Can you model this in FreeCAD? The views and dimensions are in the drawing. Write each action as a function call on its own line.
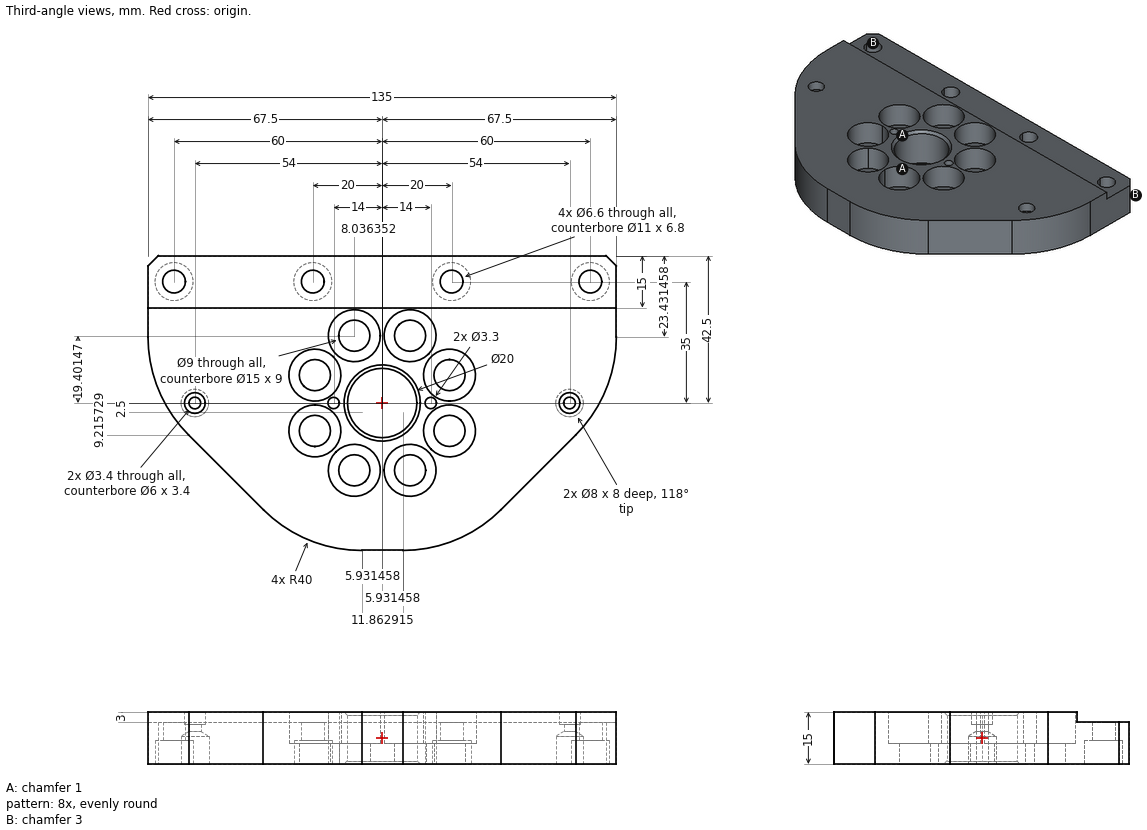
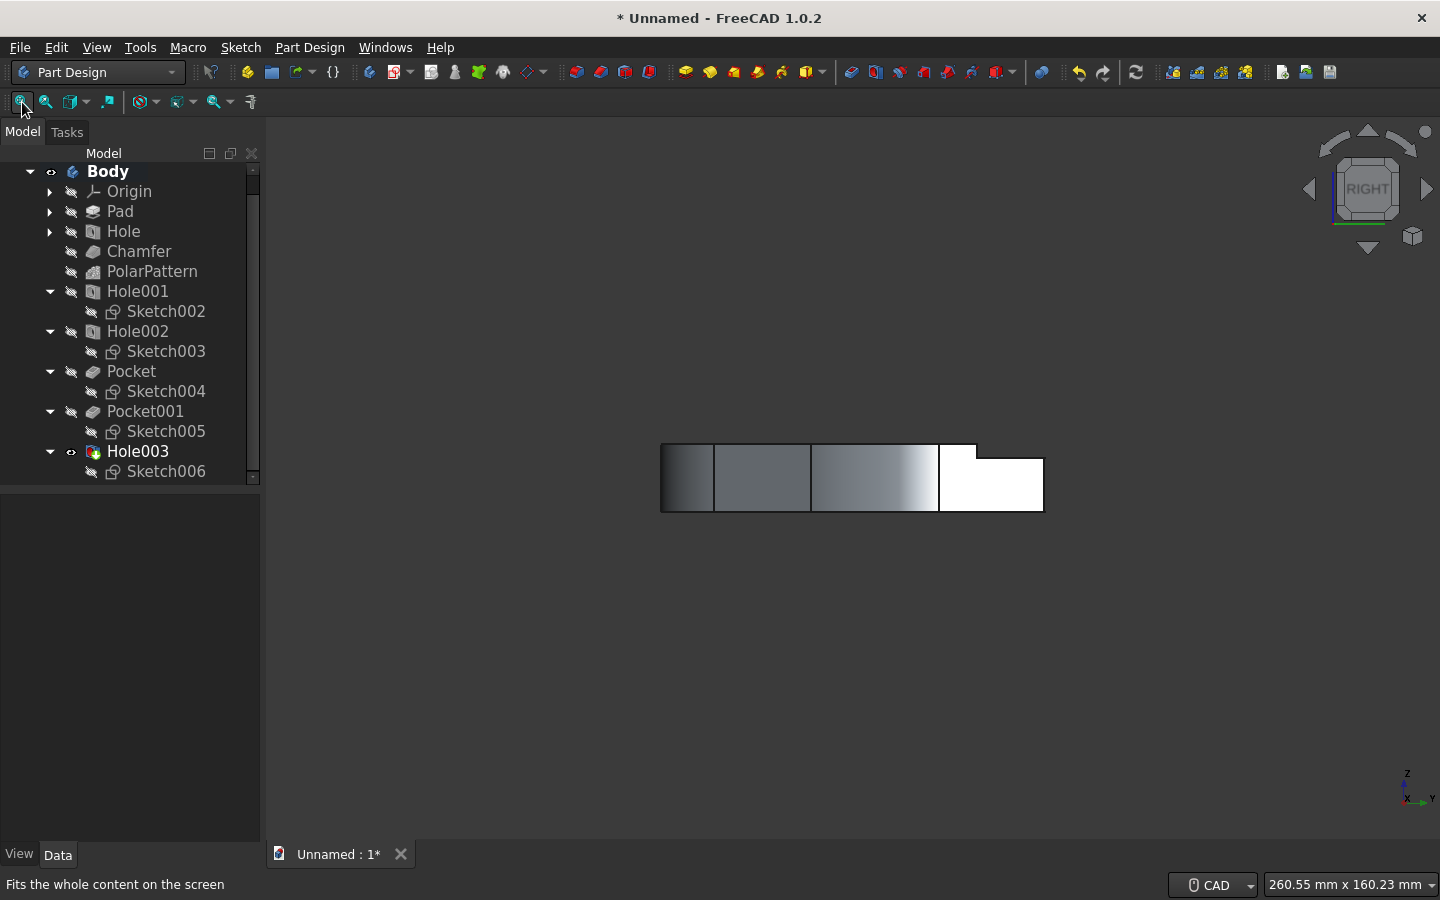
click(1045, 484)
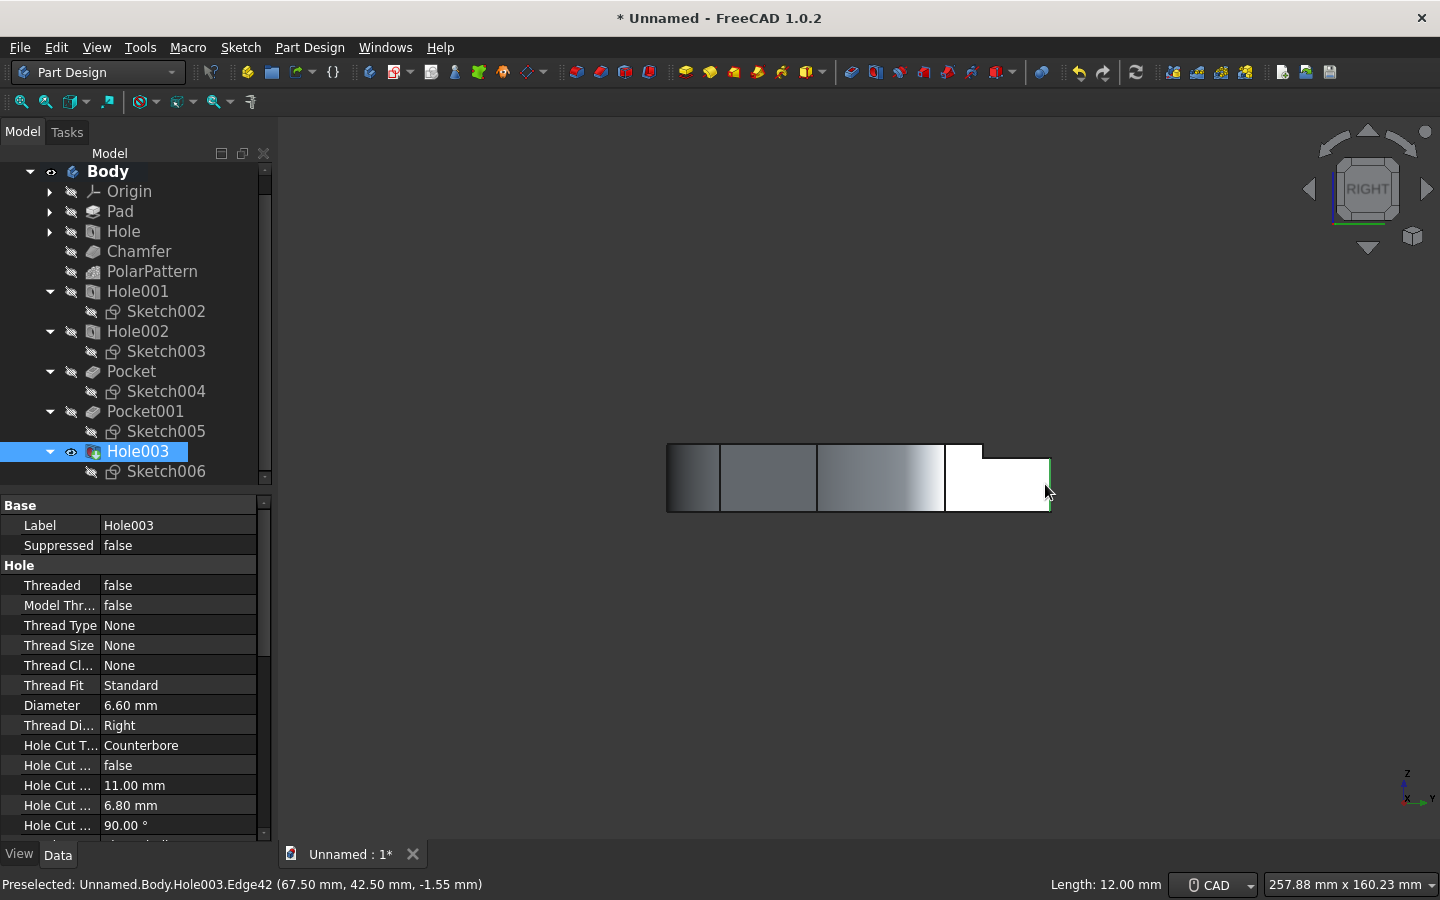
key(5)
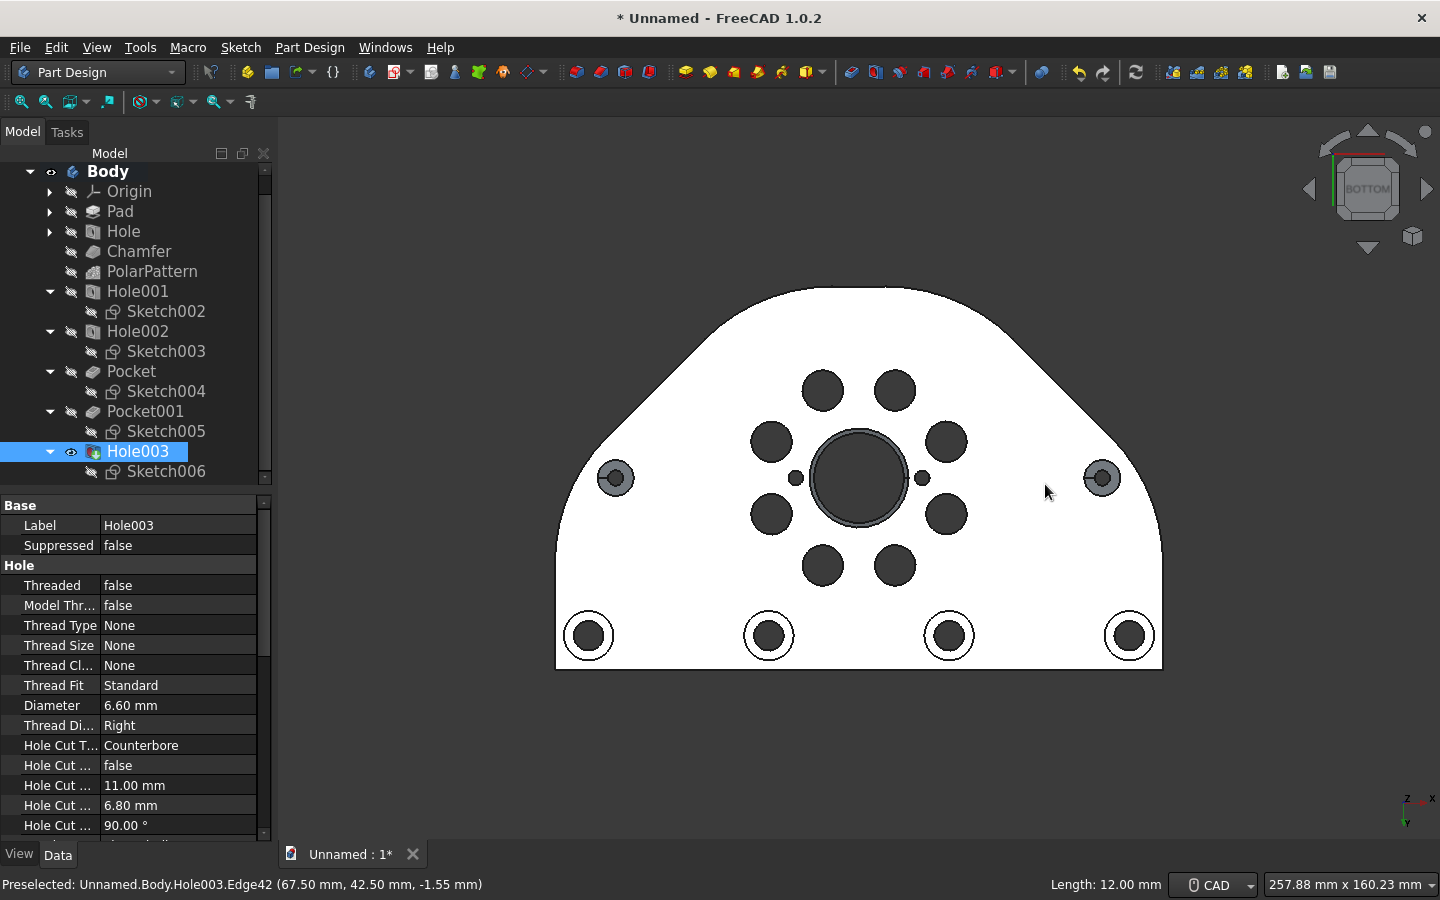
key(4)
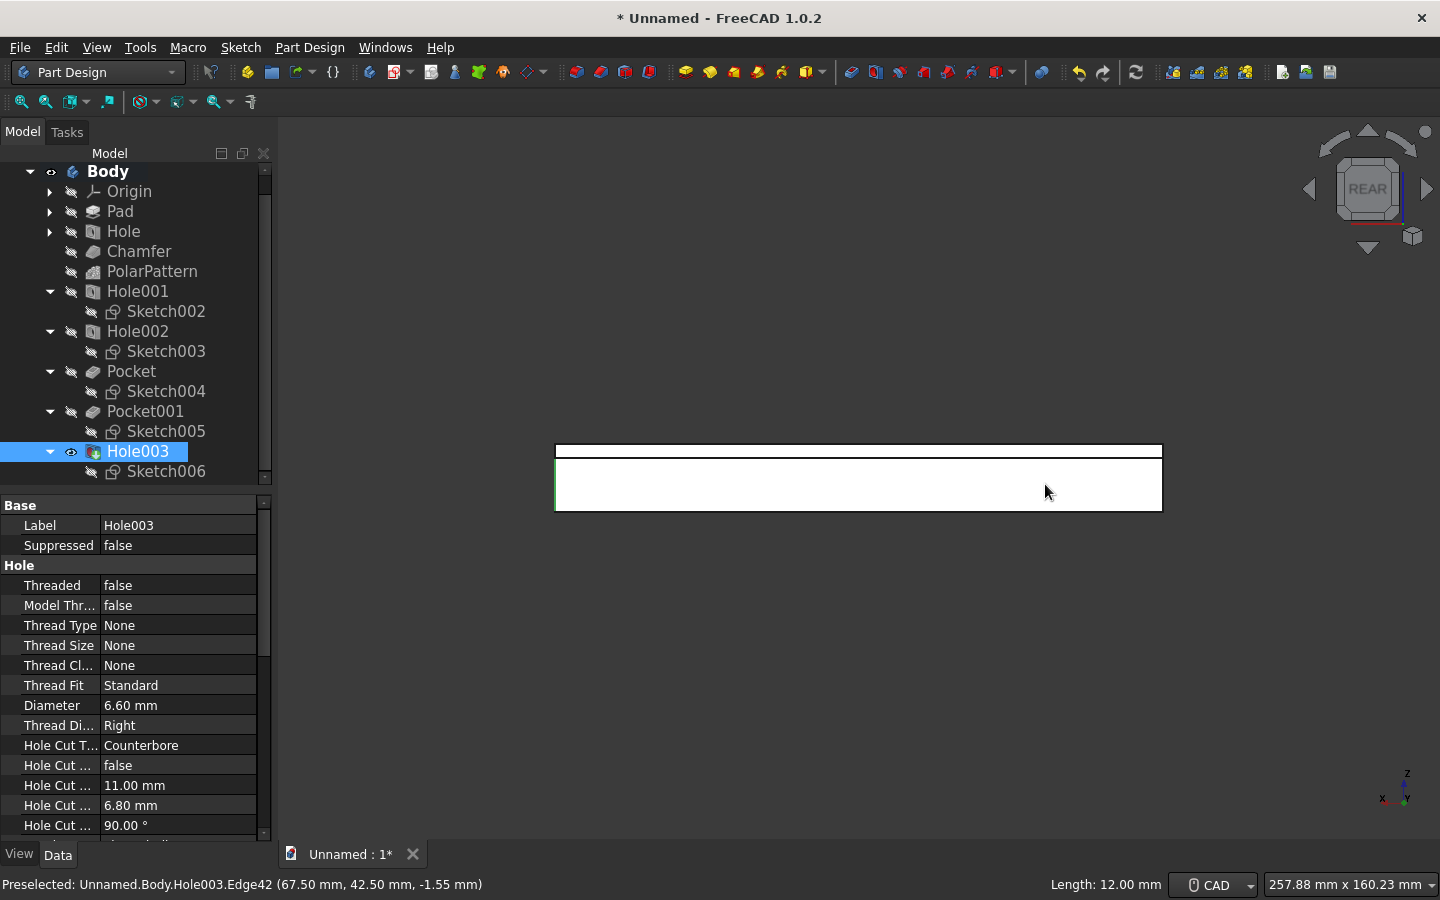
click(1163, 484, ctrl)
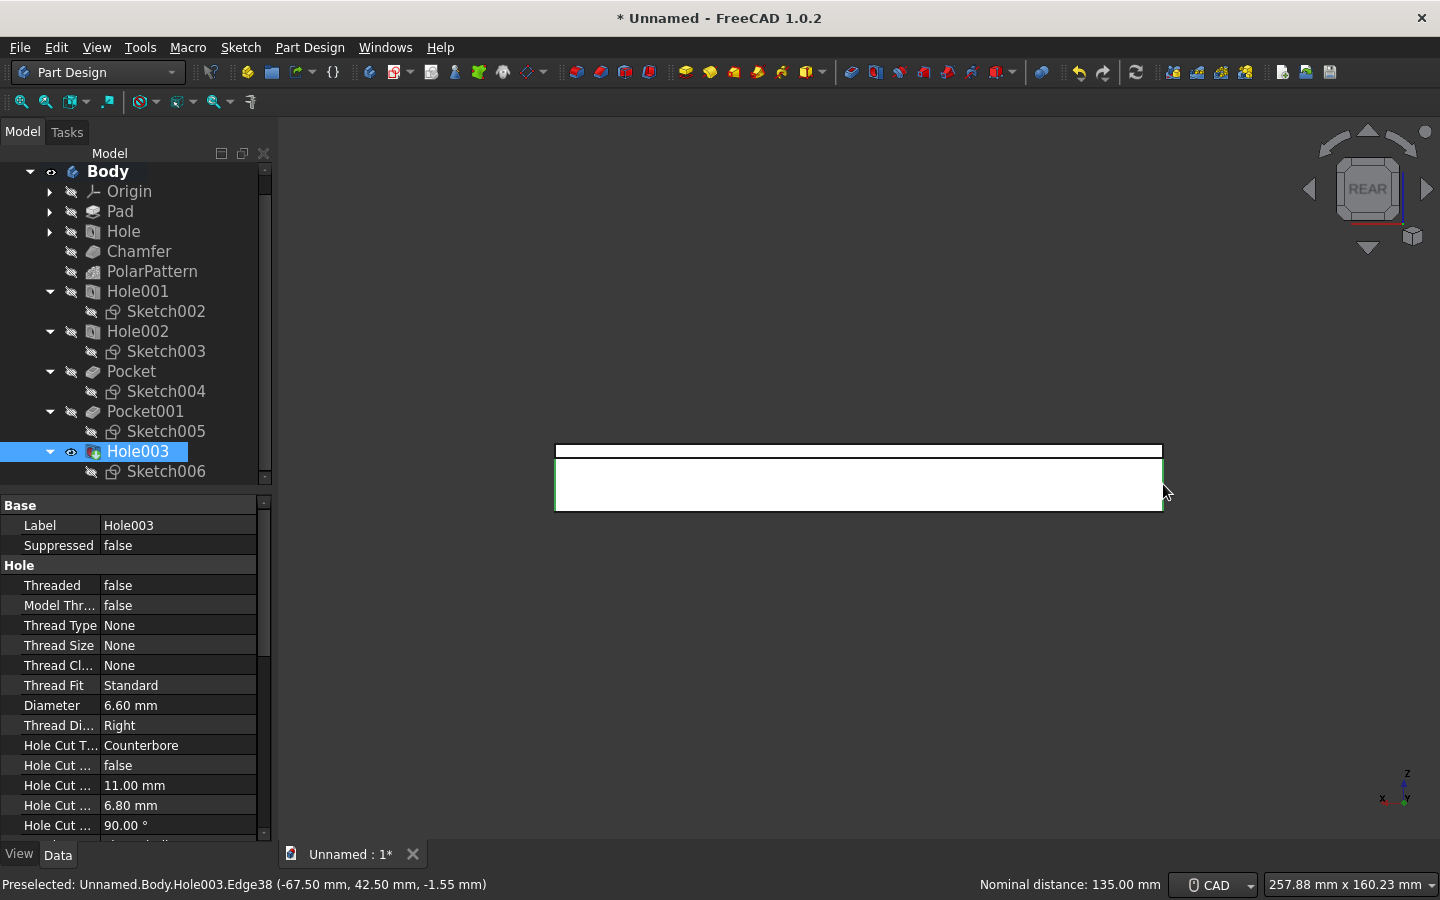
click(602, 72)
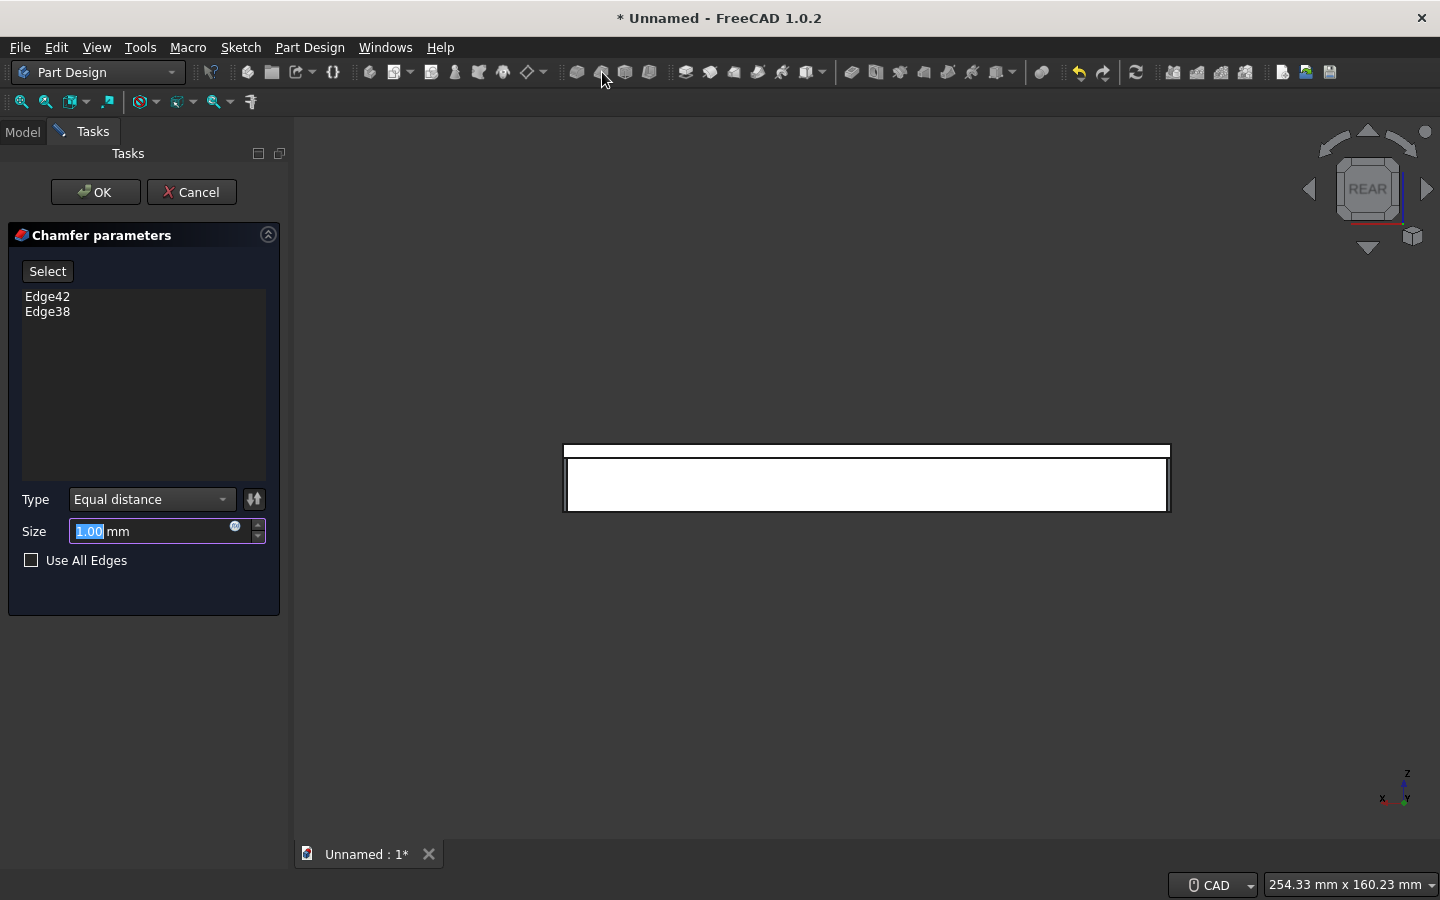
text(3)
key(Tab)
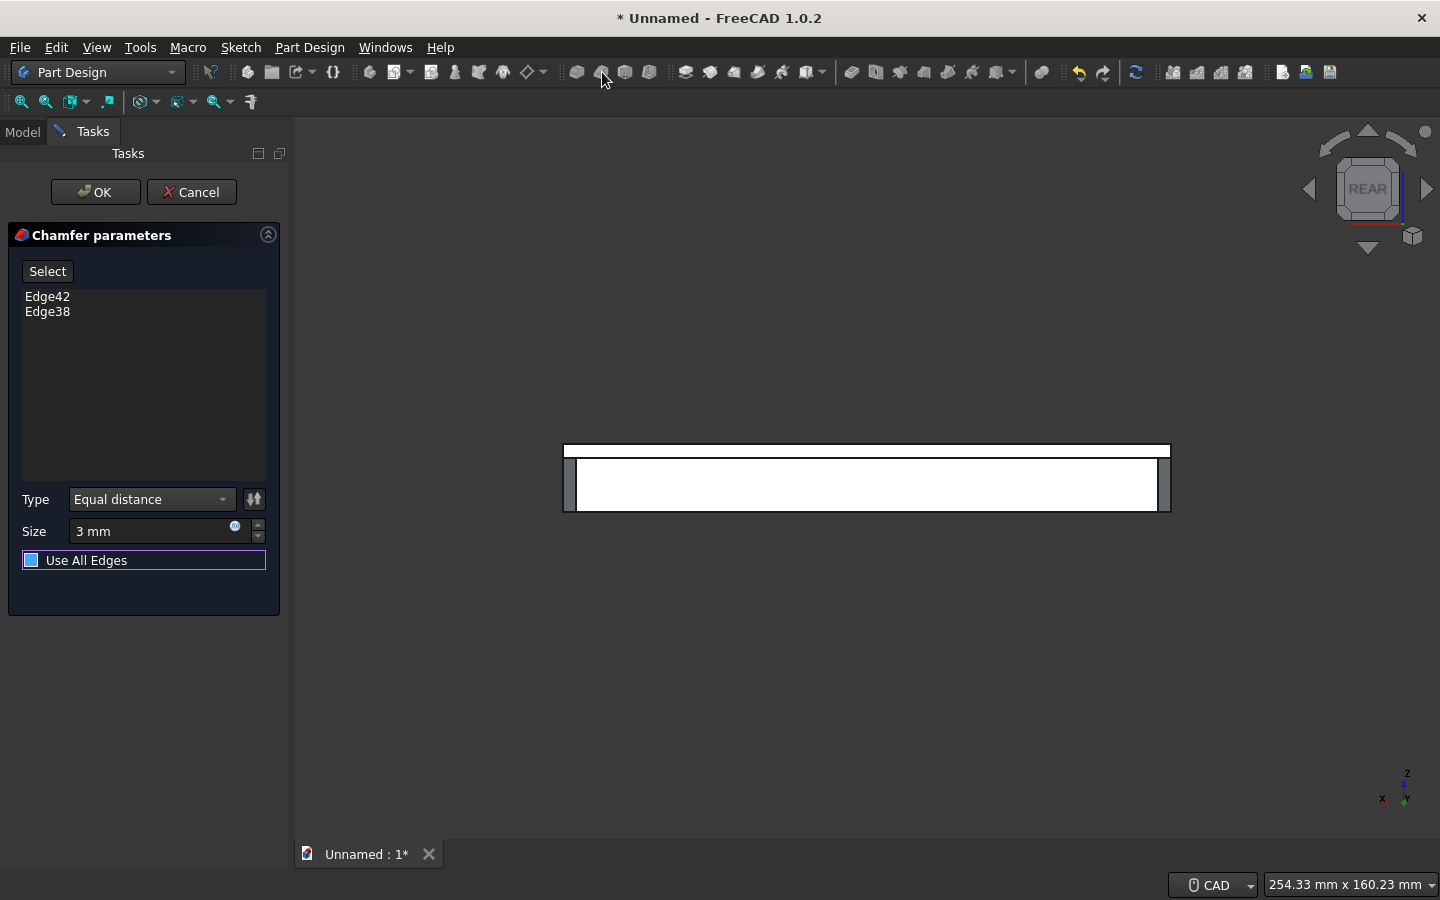
click(96, 192)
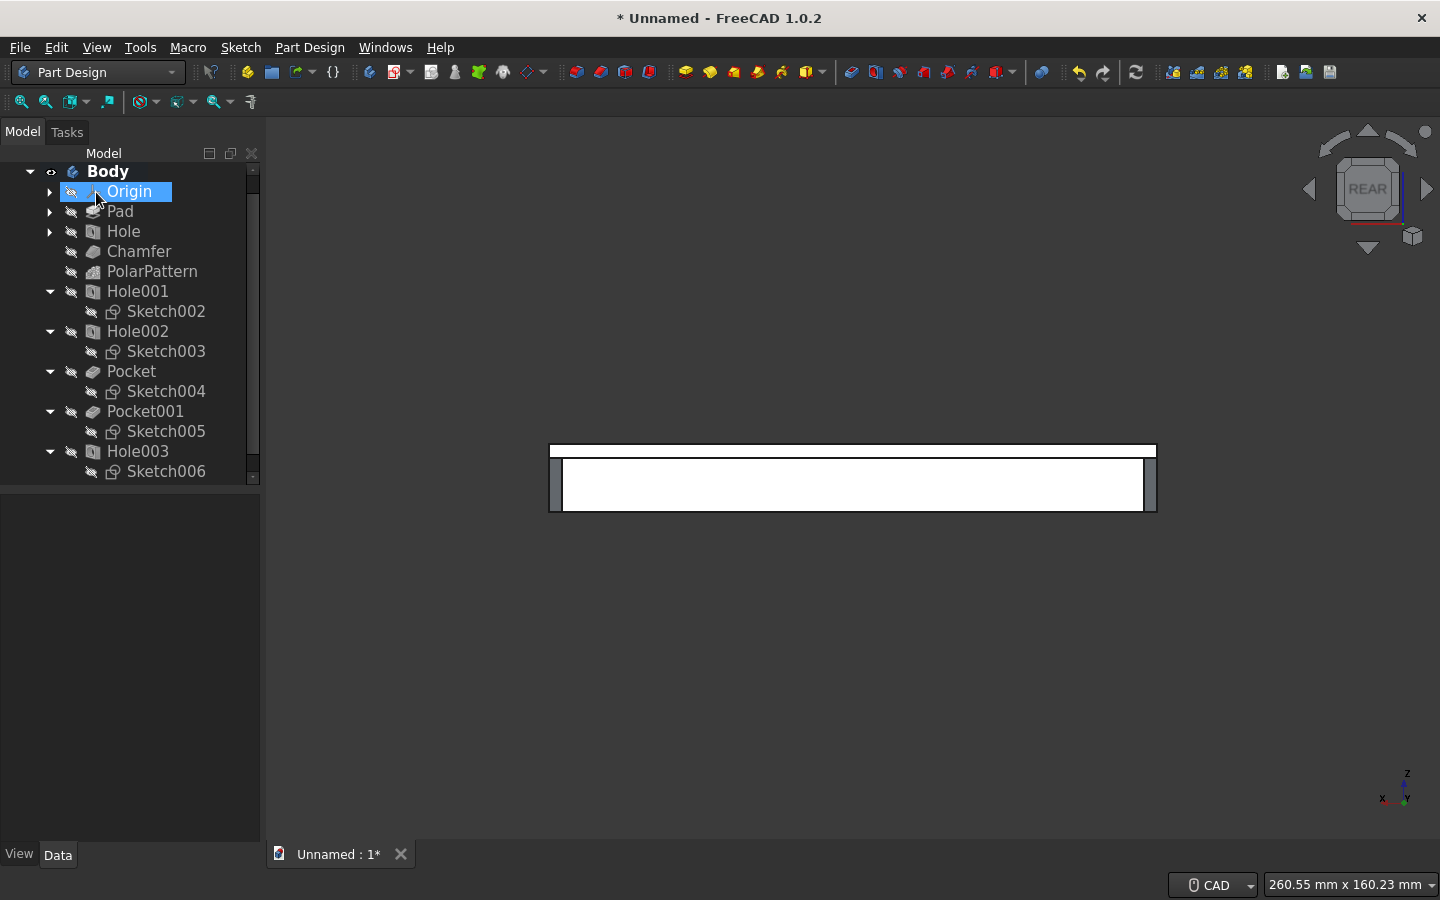
key(0)